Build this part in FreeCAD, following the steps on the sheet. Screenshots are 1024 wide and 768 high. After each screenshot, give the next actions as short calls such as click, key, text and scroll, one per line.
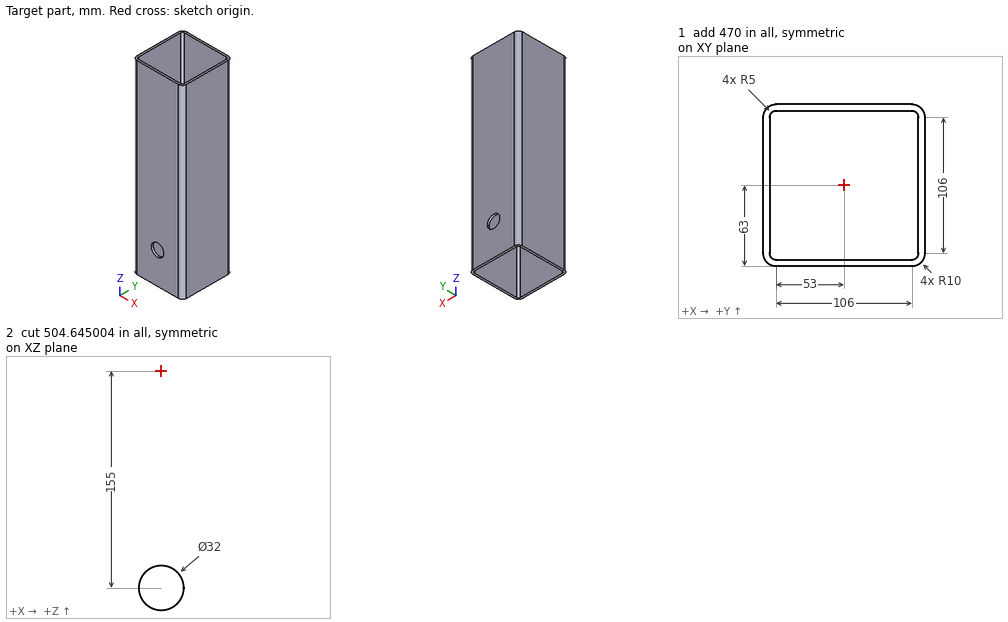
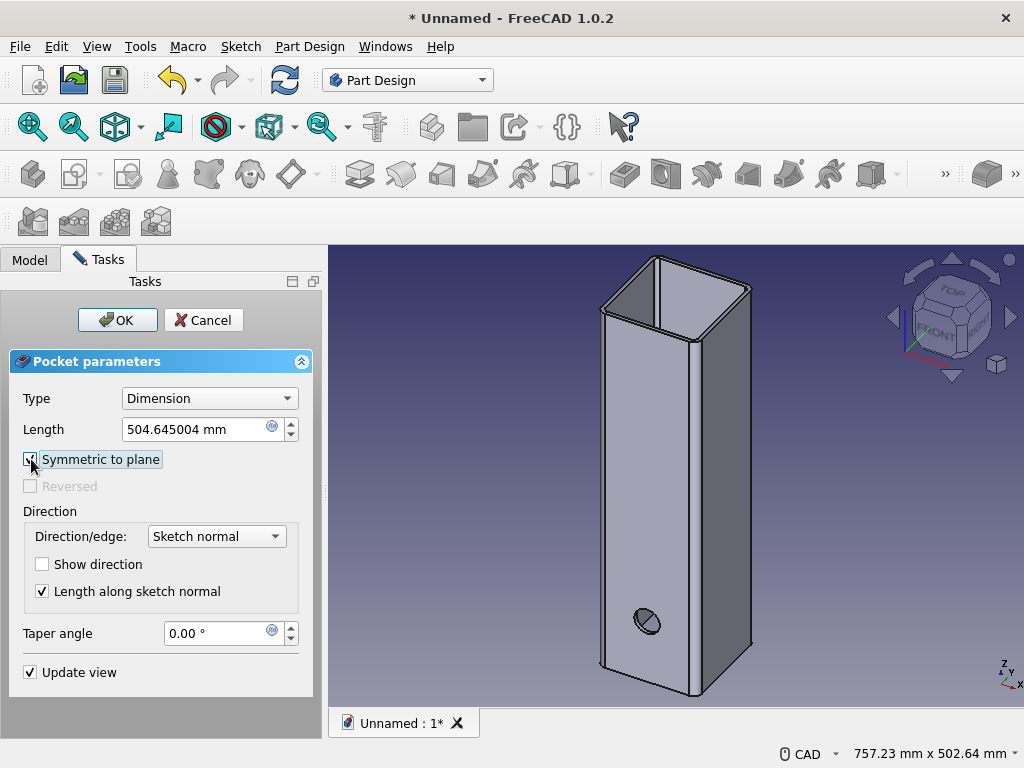
click(118, 320)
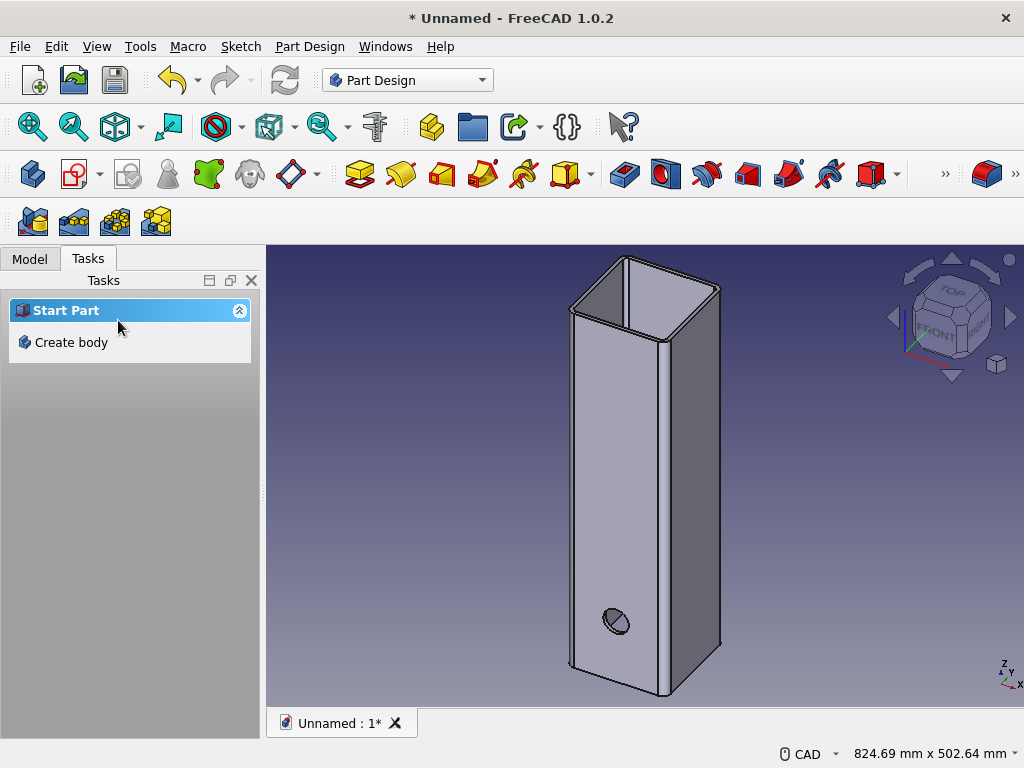
key(0)